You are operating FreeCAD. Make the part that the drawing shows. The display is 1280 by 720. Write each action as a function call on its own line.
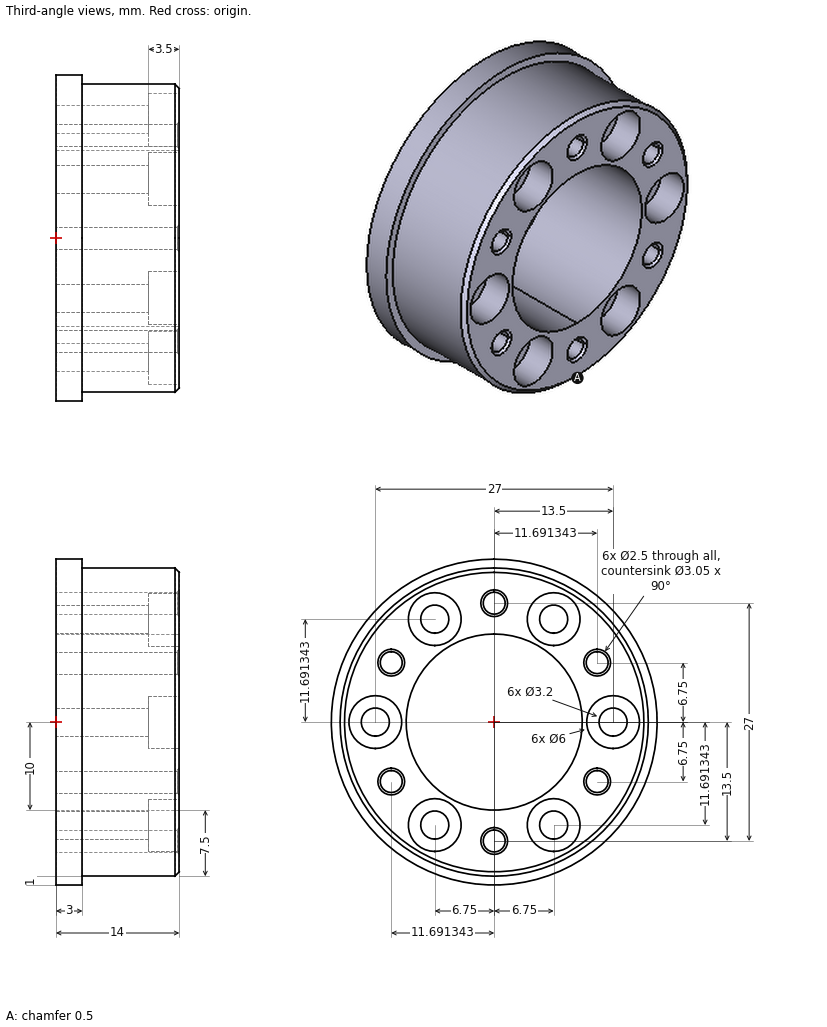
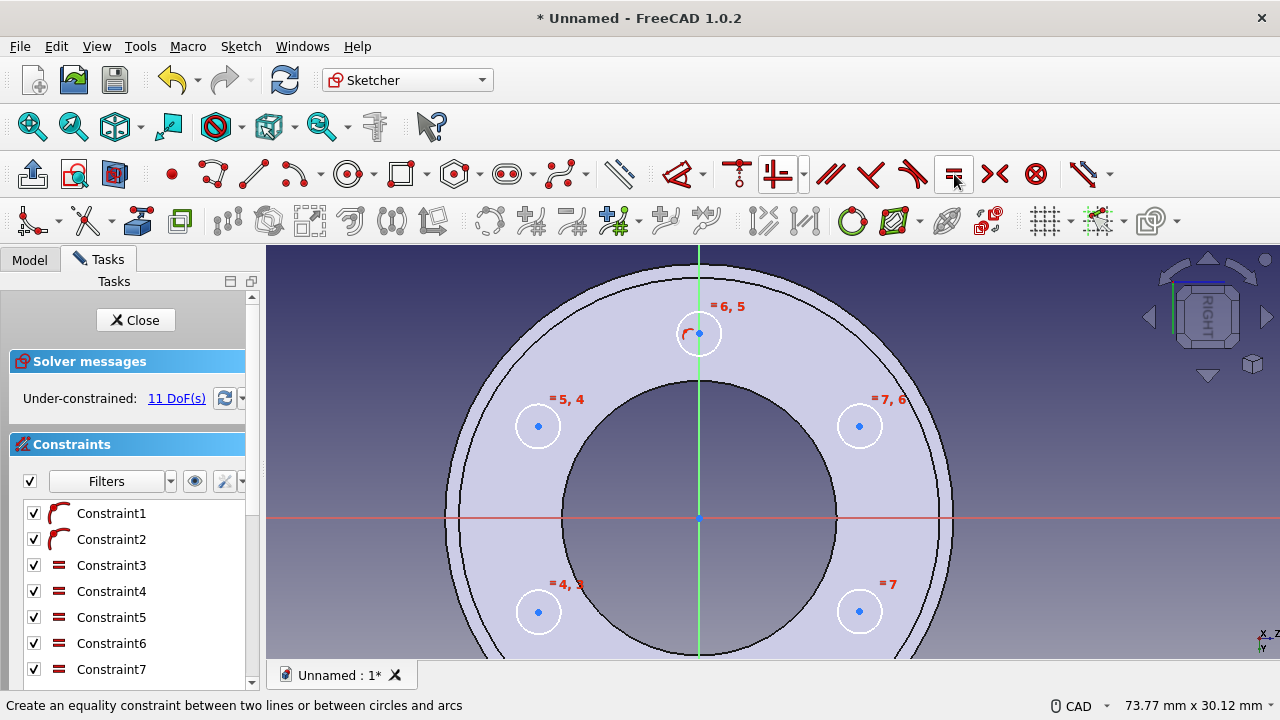
click(539, 612)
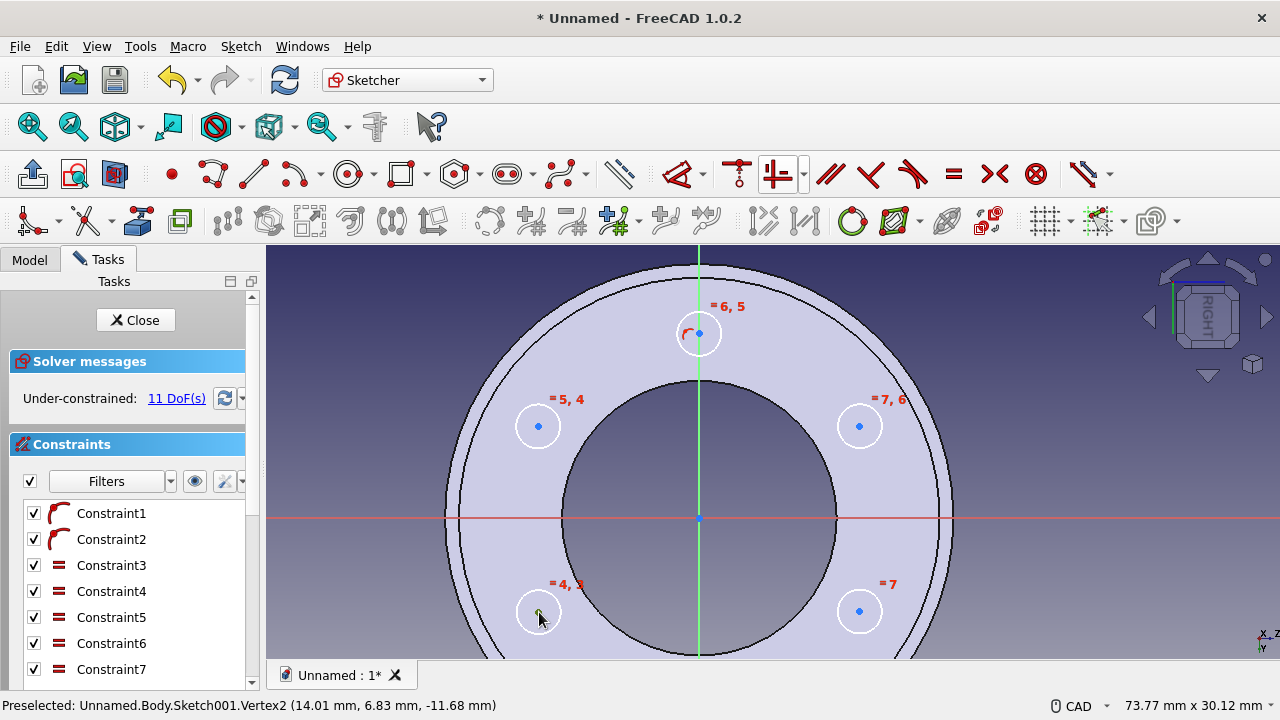
click(538, 426)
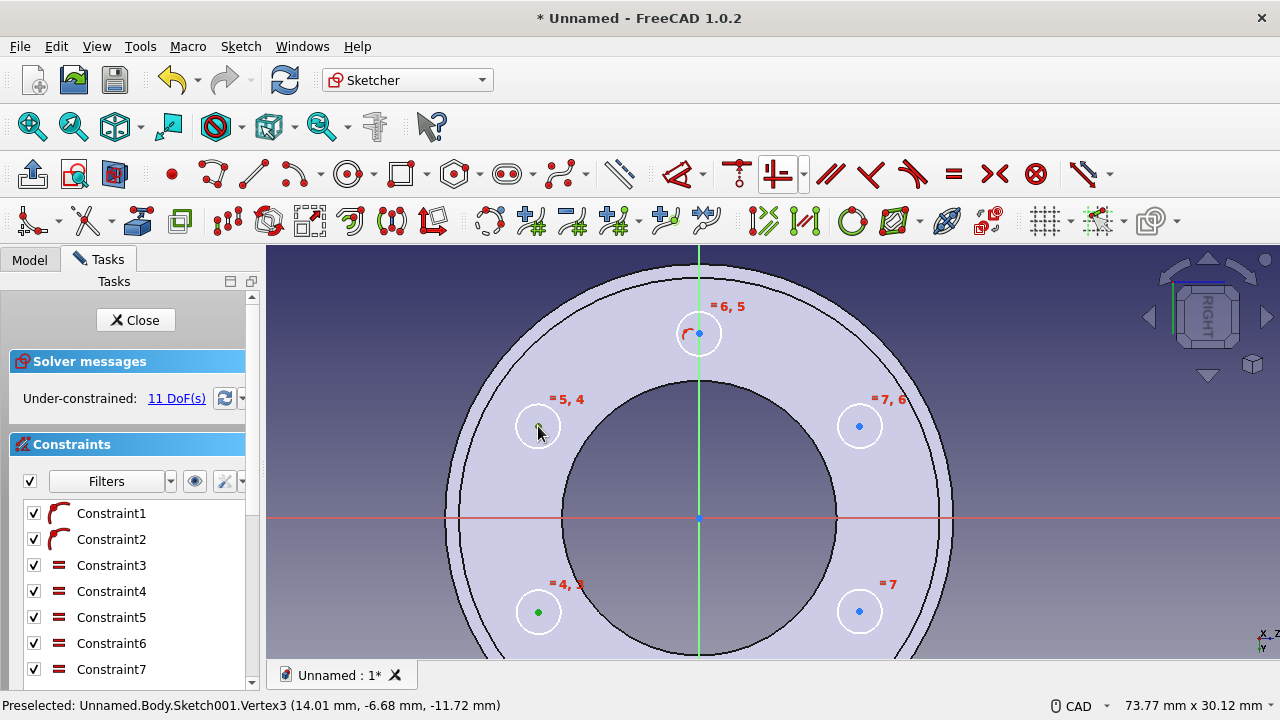
click(804, 174)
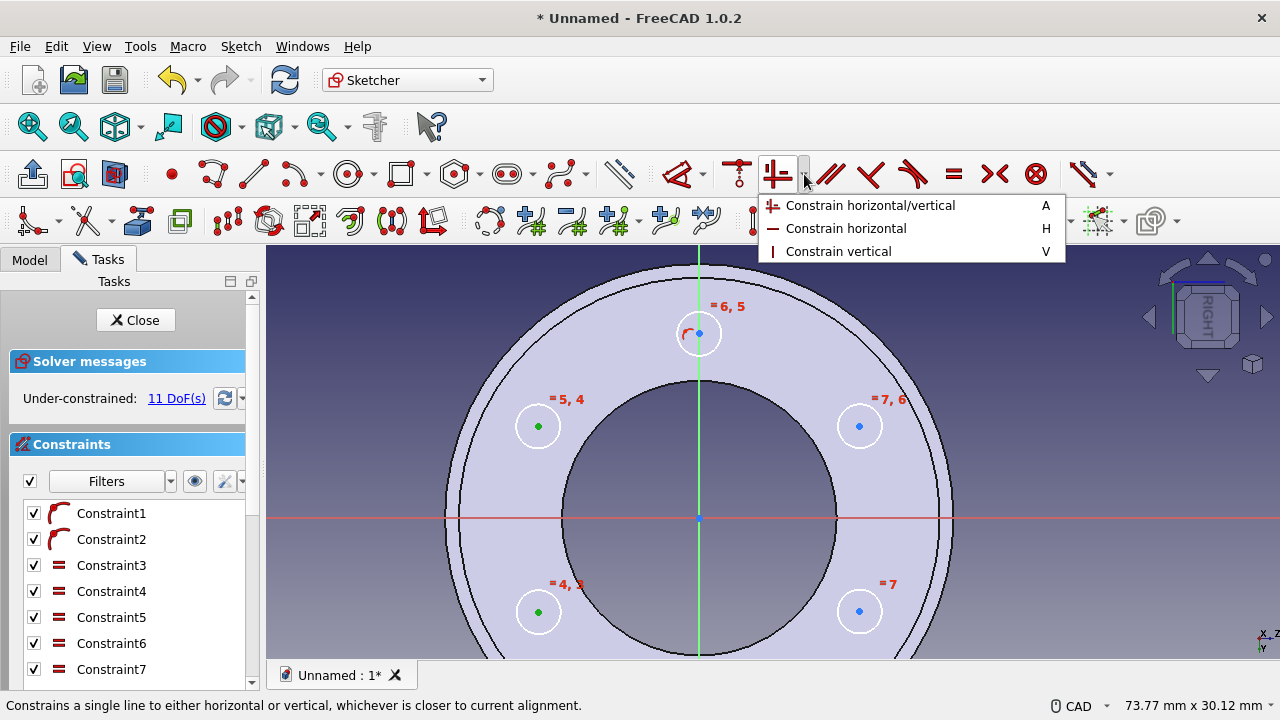
click(912, 252)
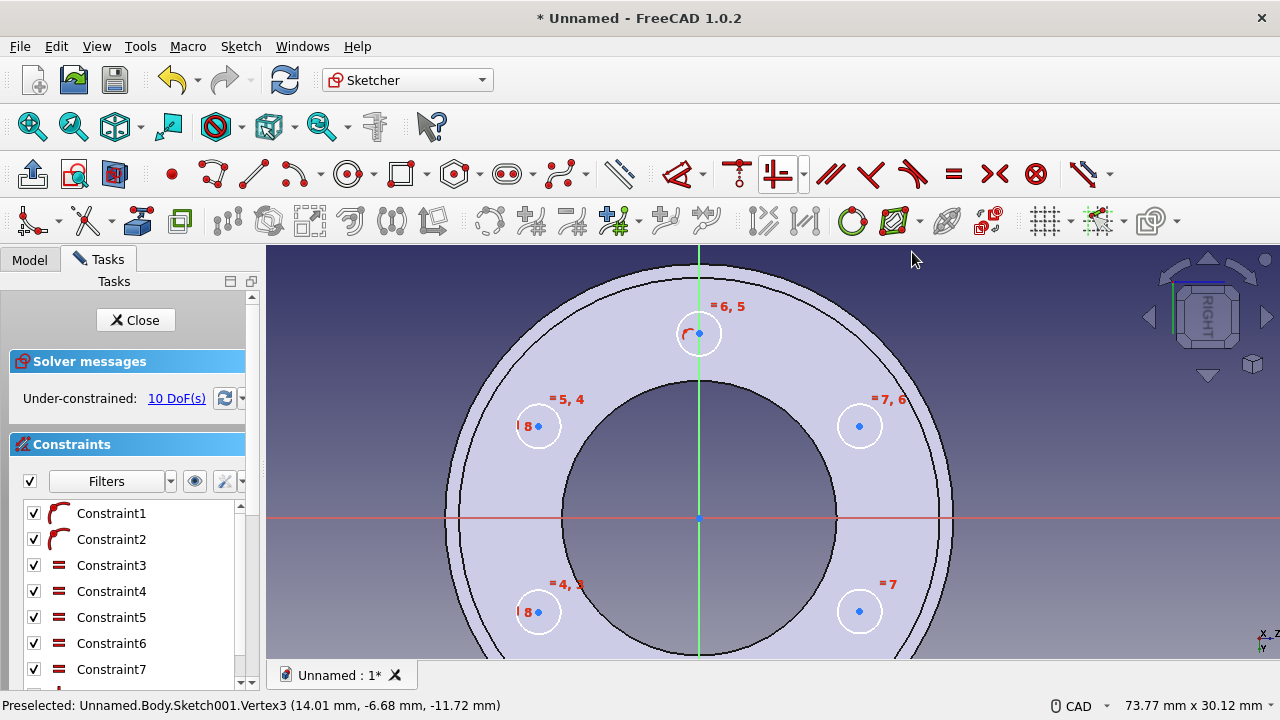
click(539, 426)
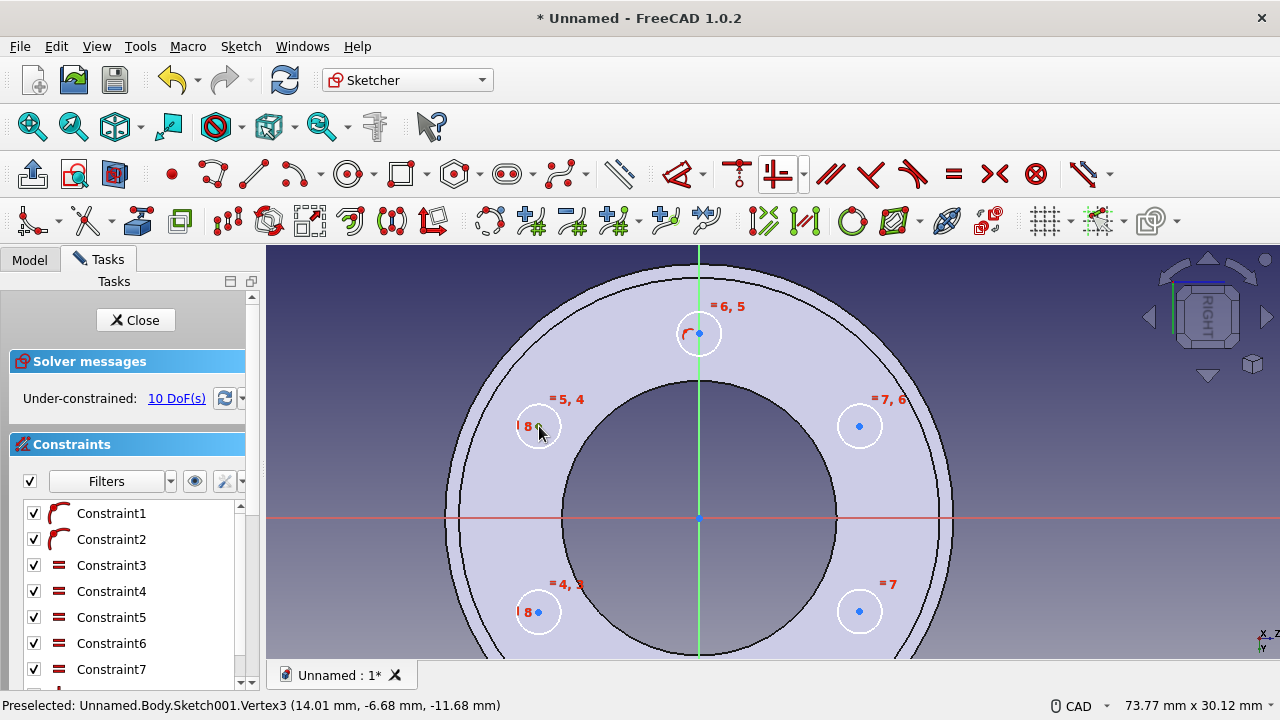
click(860, 426)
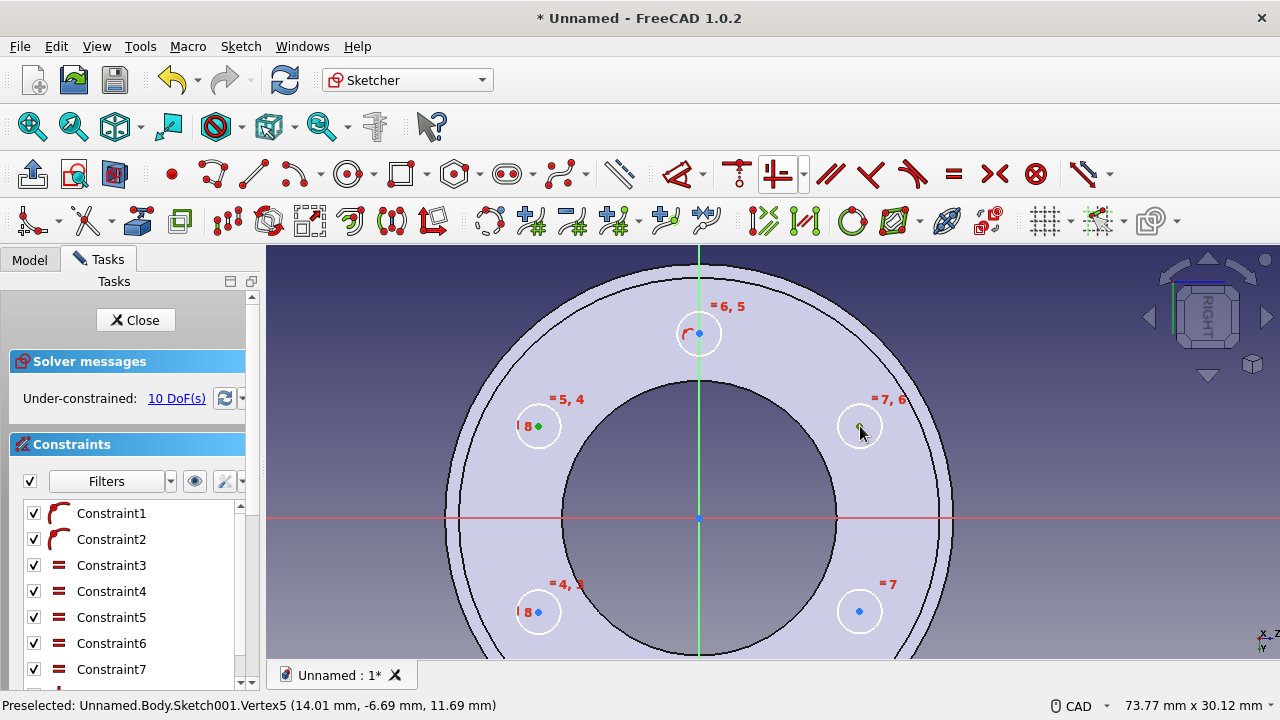
key(h)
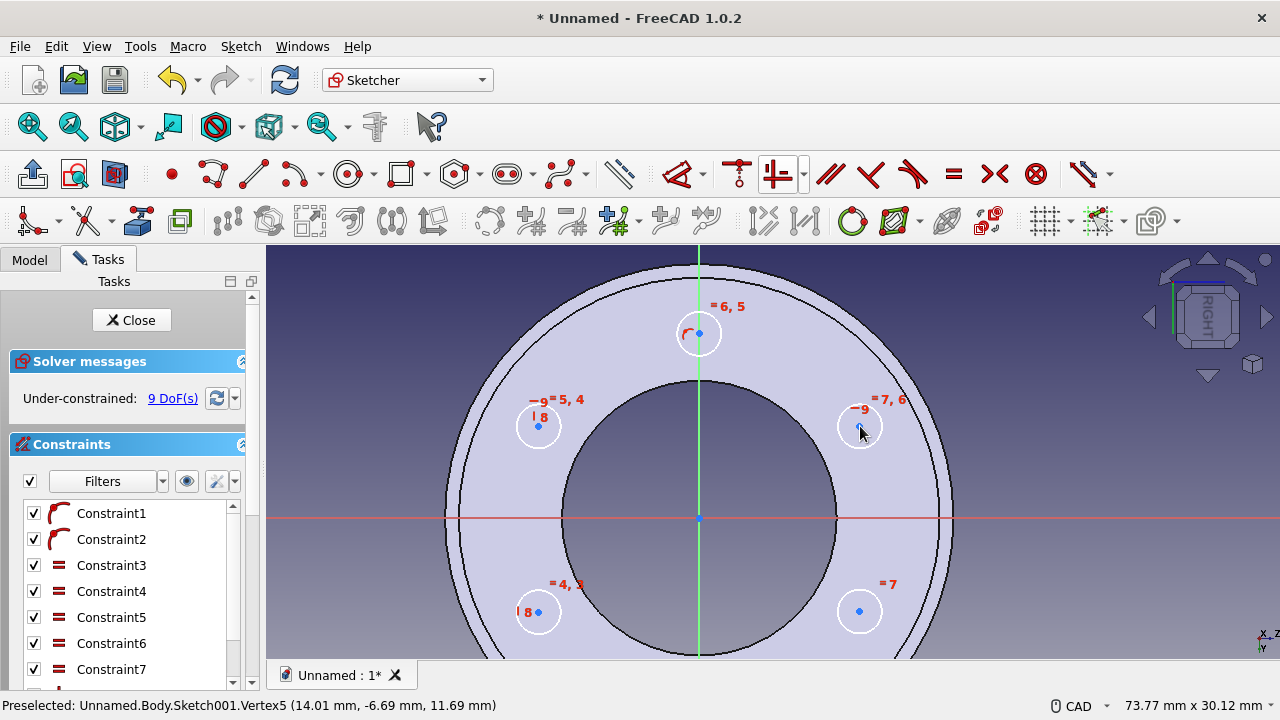
click(860, 426)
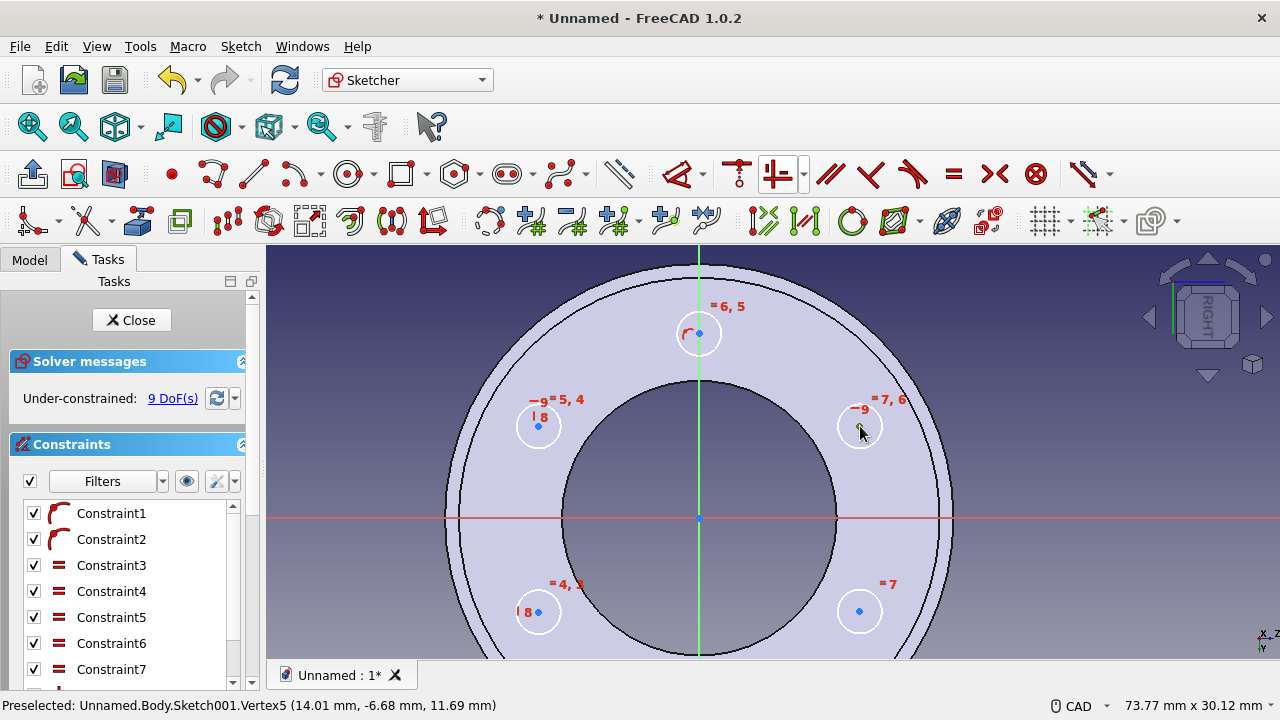
click(860, 612)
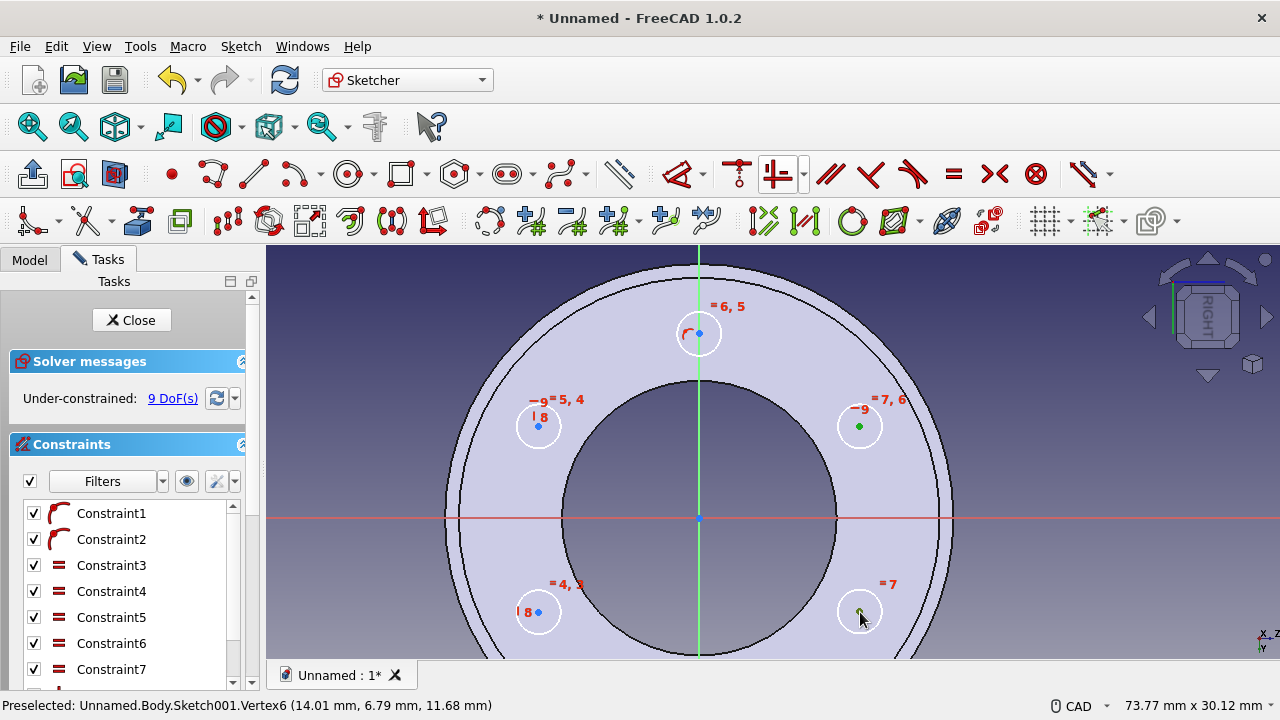
click(804, 174)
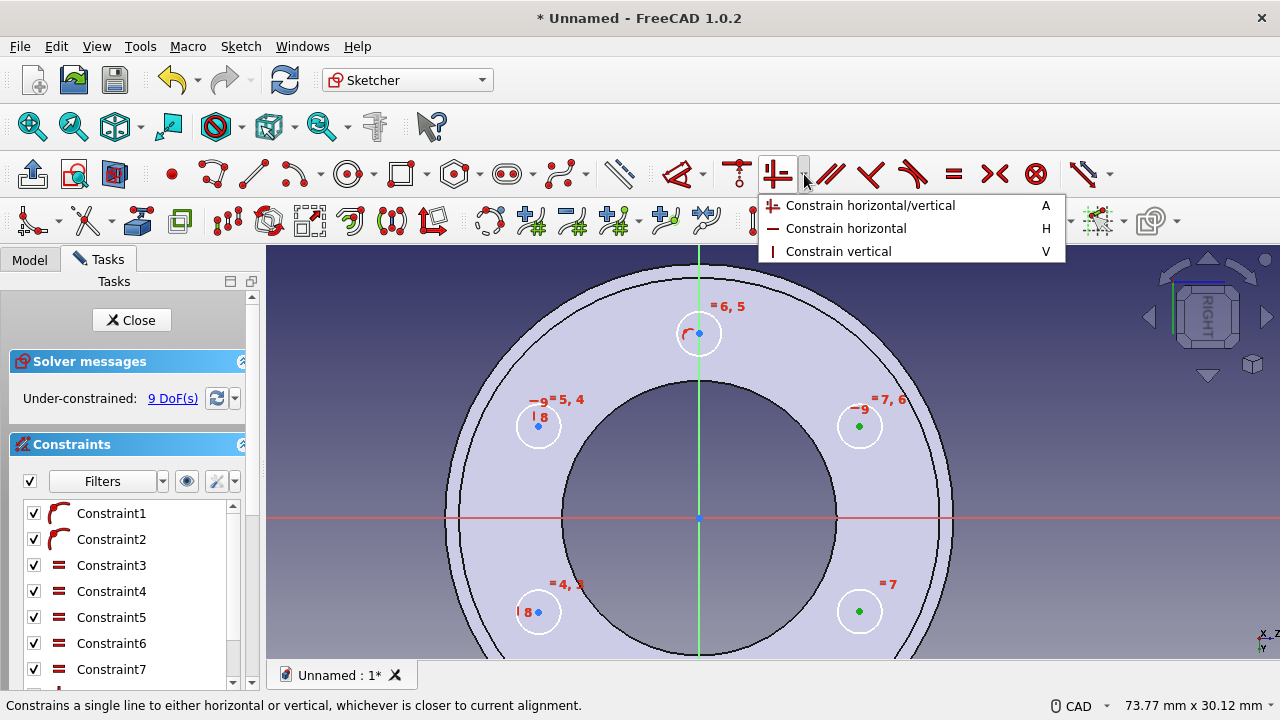
click(912, 252)